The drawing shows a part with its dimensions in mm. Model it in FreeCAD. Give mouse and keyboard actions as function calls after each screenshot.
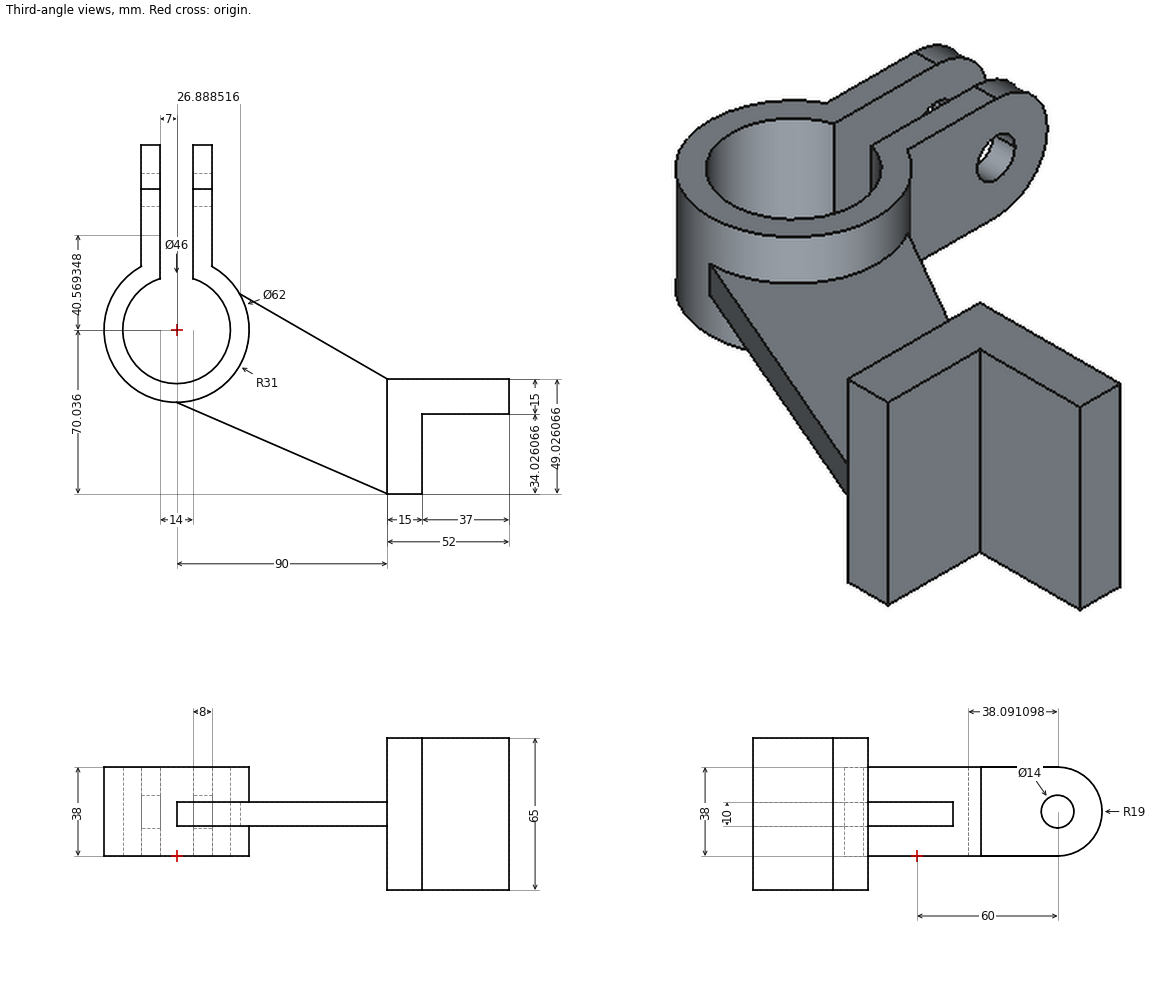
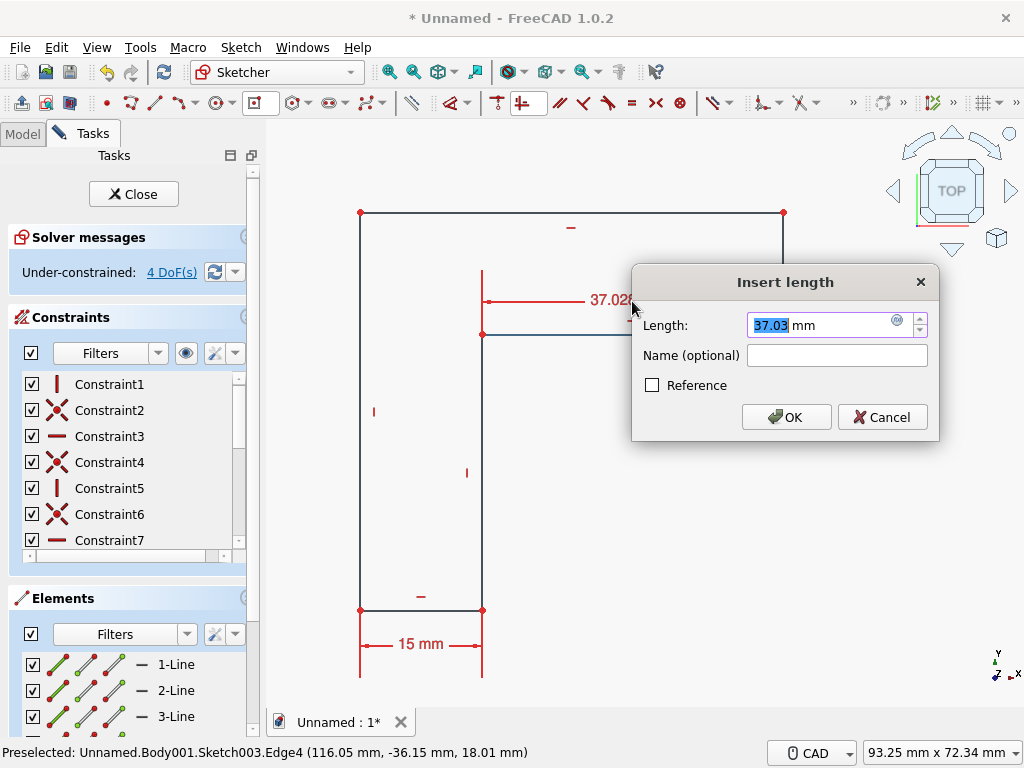
text(37)
key(Return)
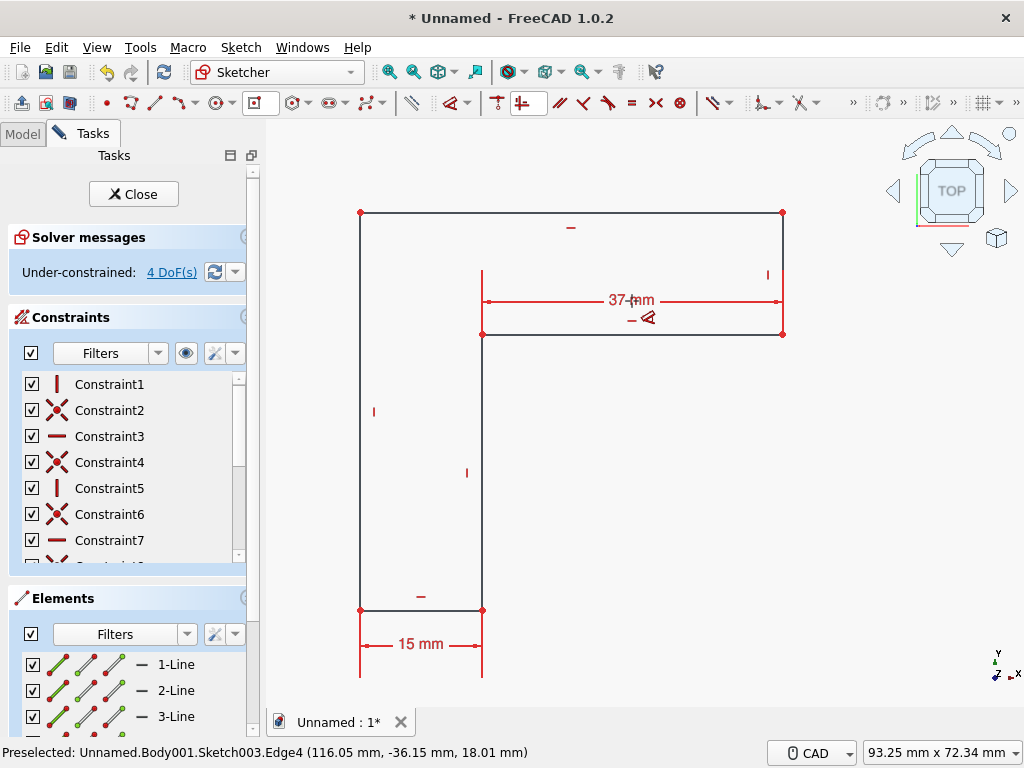
click(783, 298)
click(817, 274)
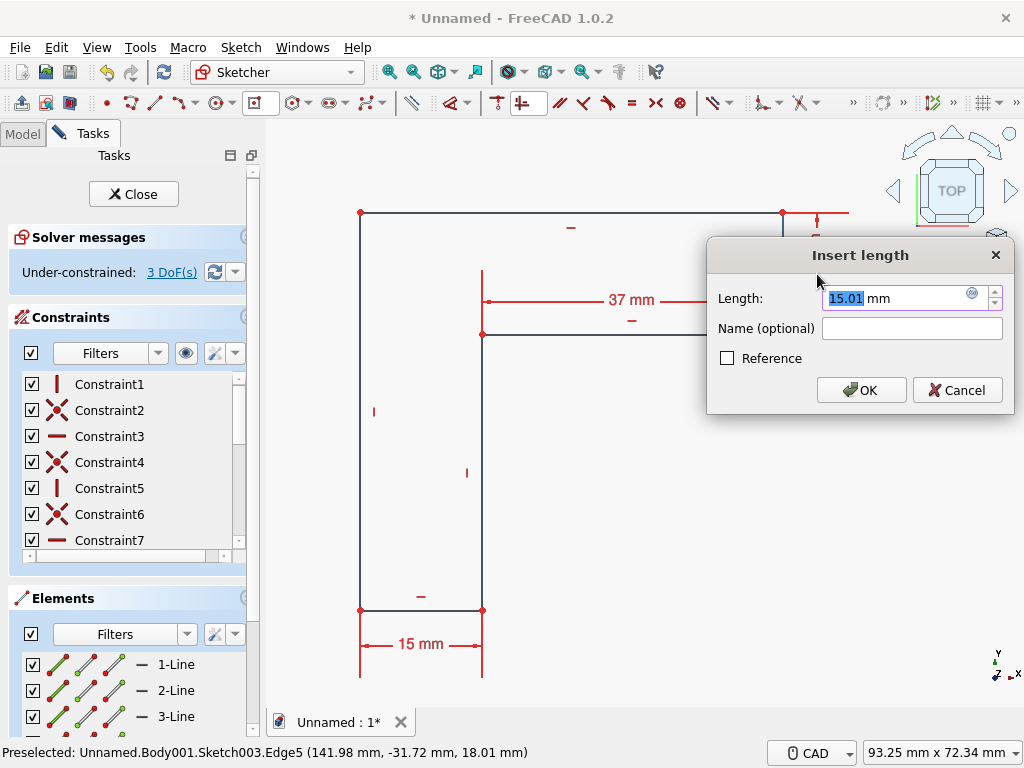
text(15)
key(Return)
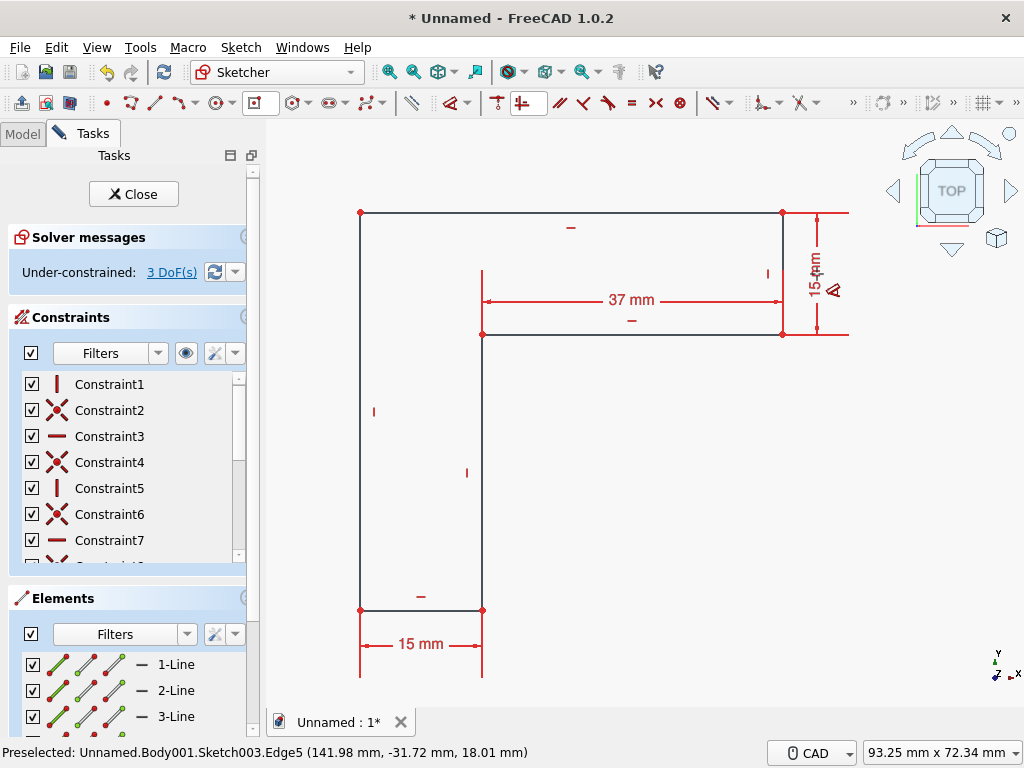
click(360, 213)
click(327, 247)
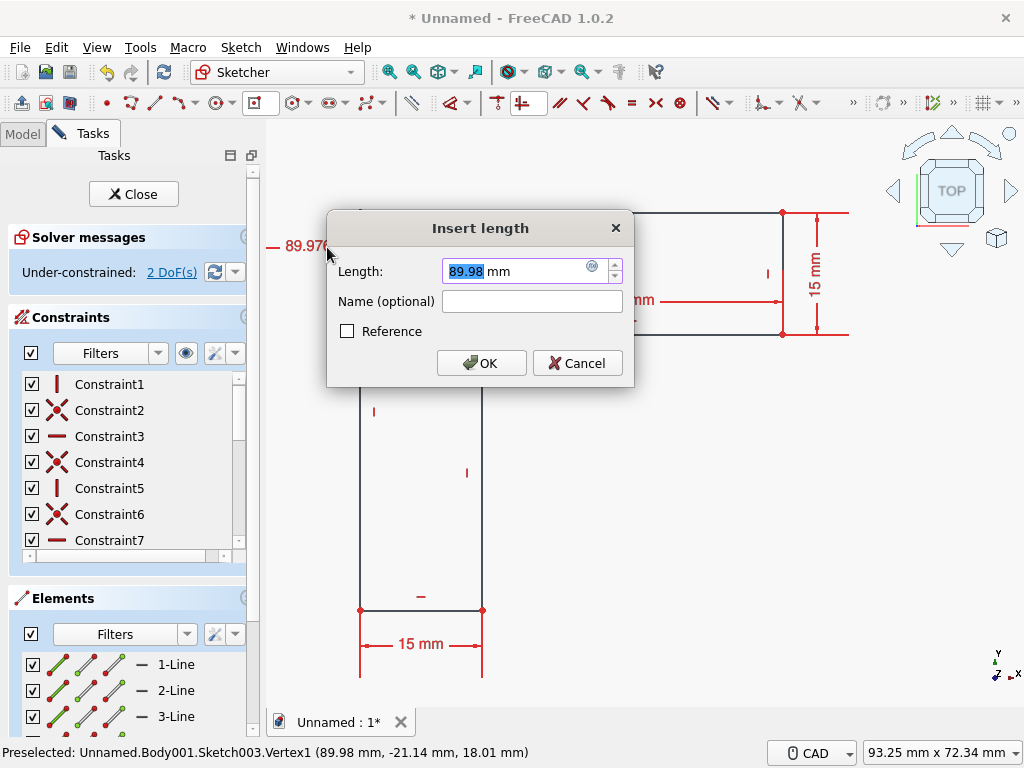
text(90)
key(Return)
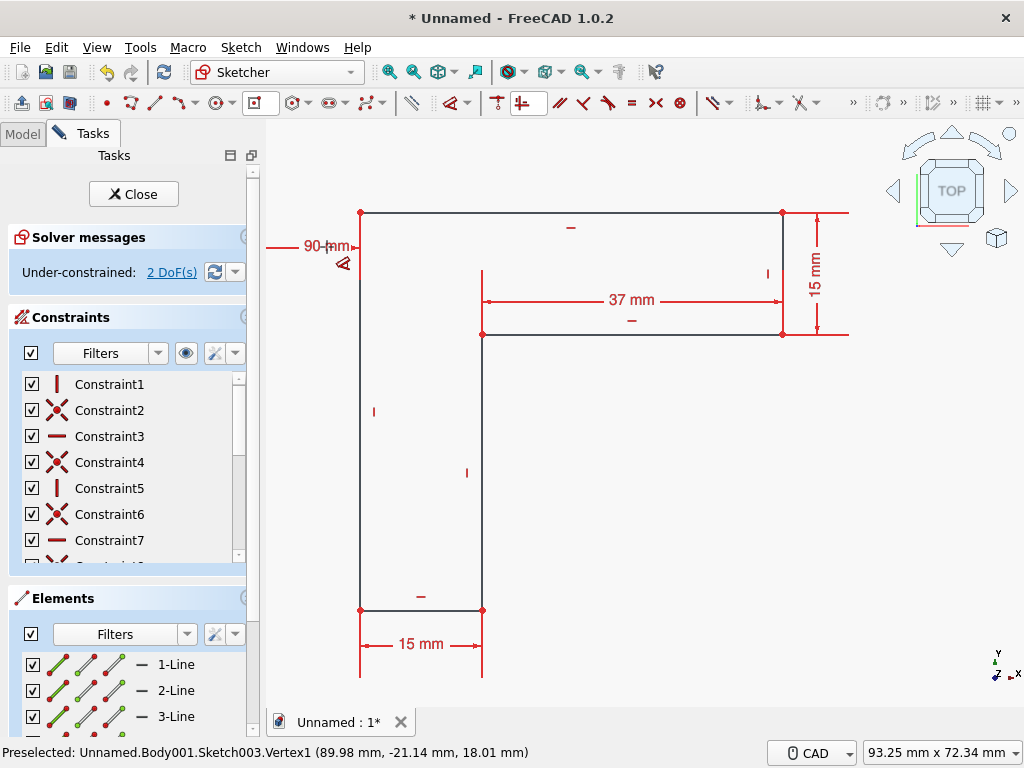
click(360, 611)
click(394, 379)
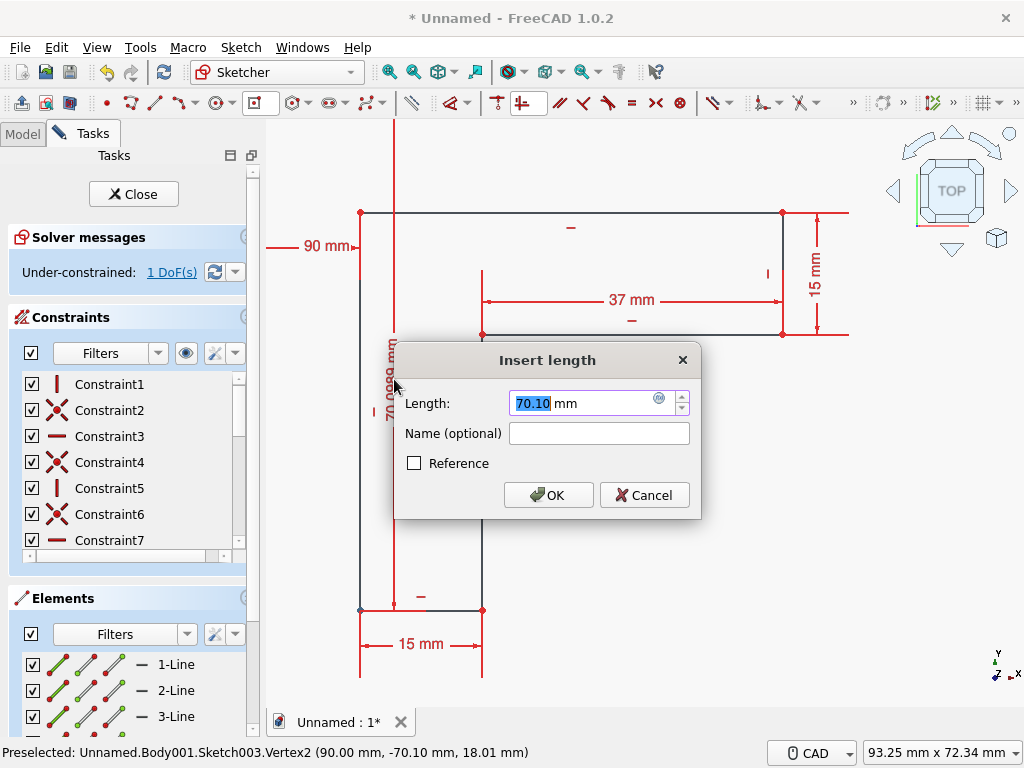
text(70.036)
key(Return)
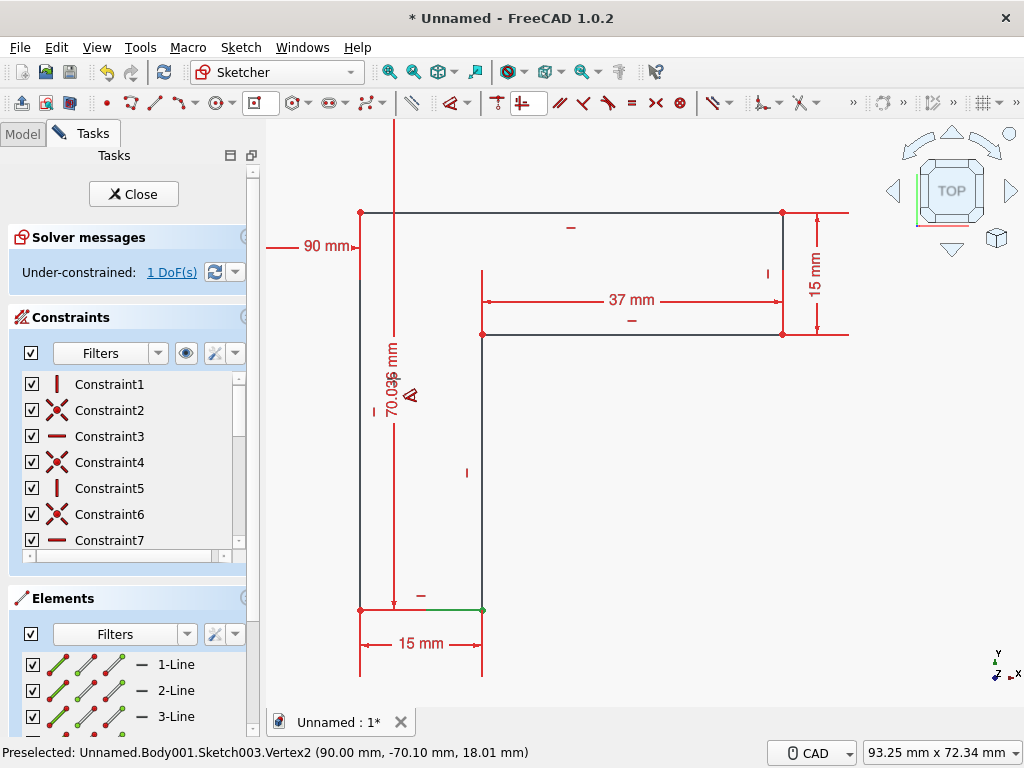
click(360, 332)
click(326, 412)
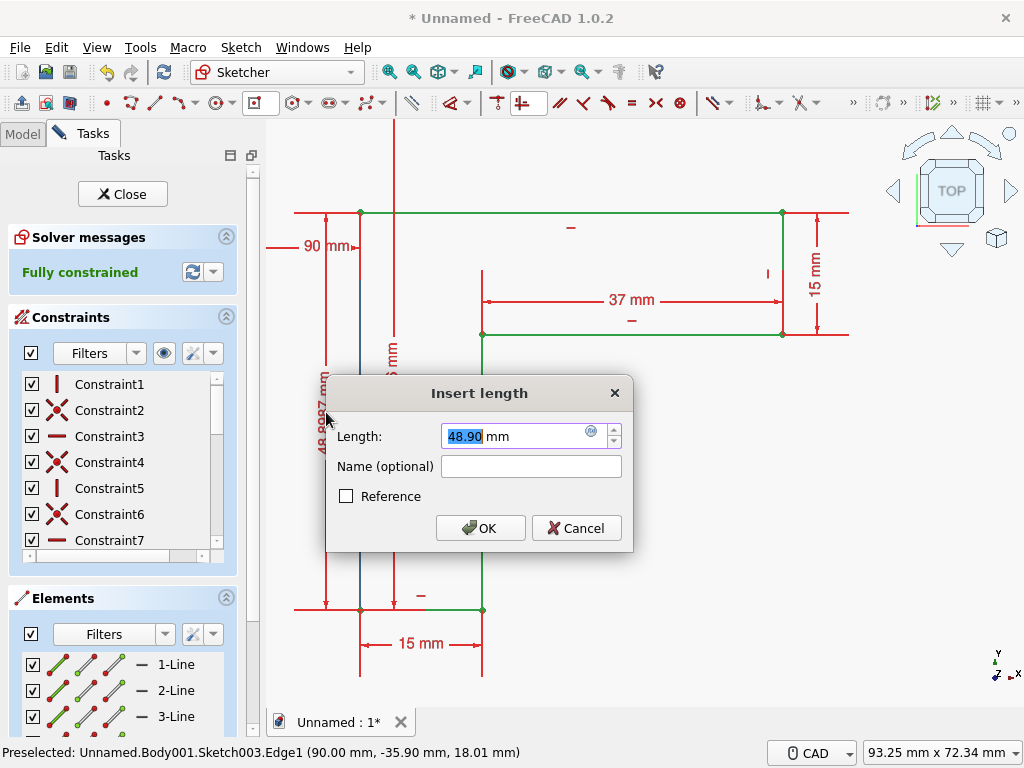
text(49.026066)
key(Return)
key(Escape)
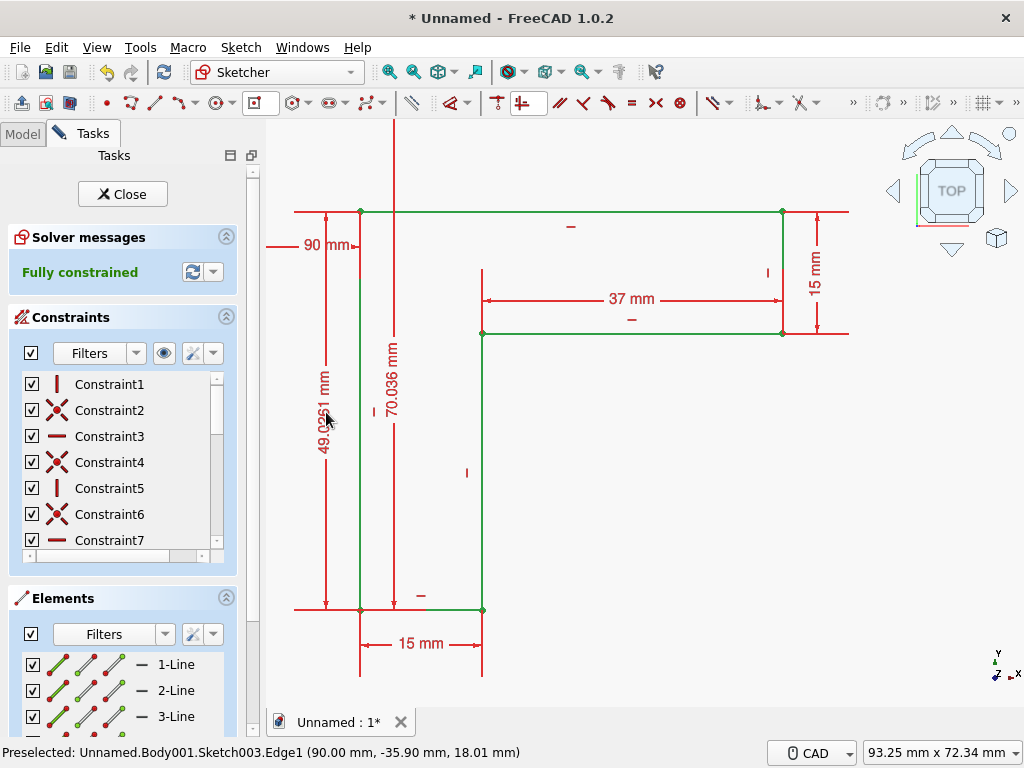
click(123, 194)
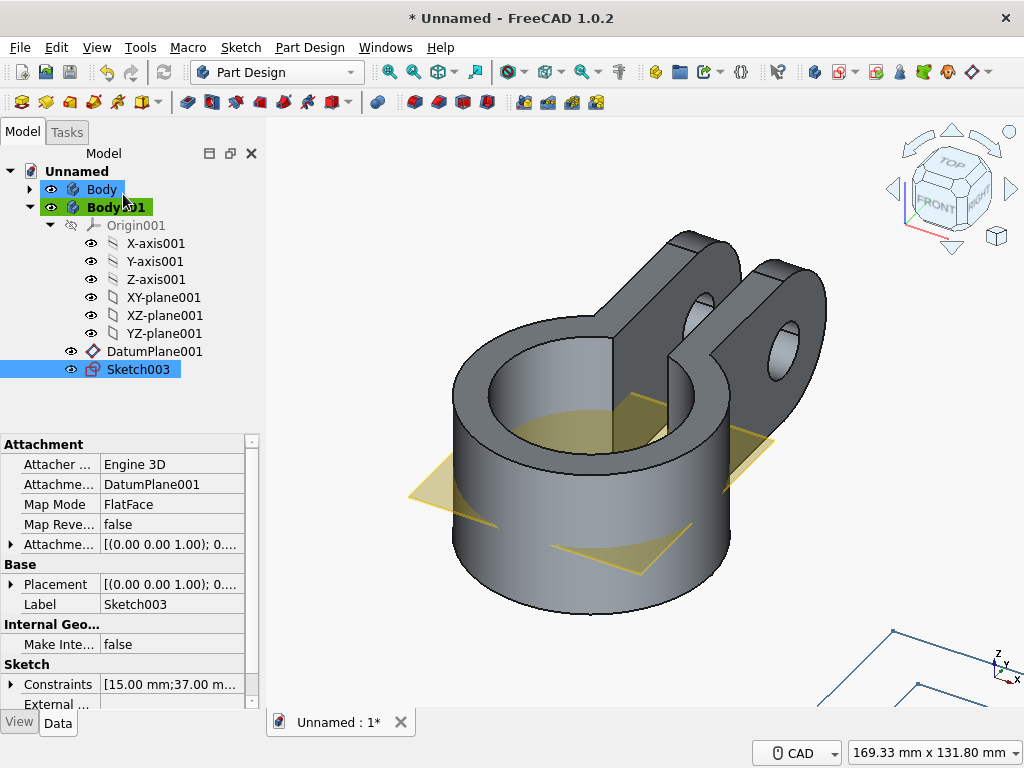
click(22, 102)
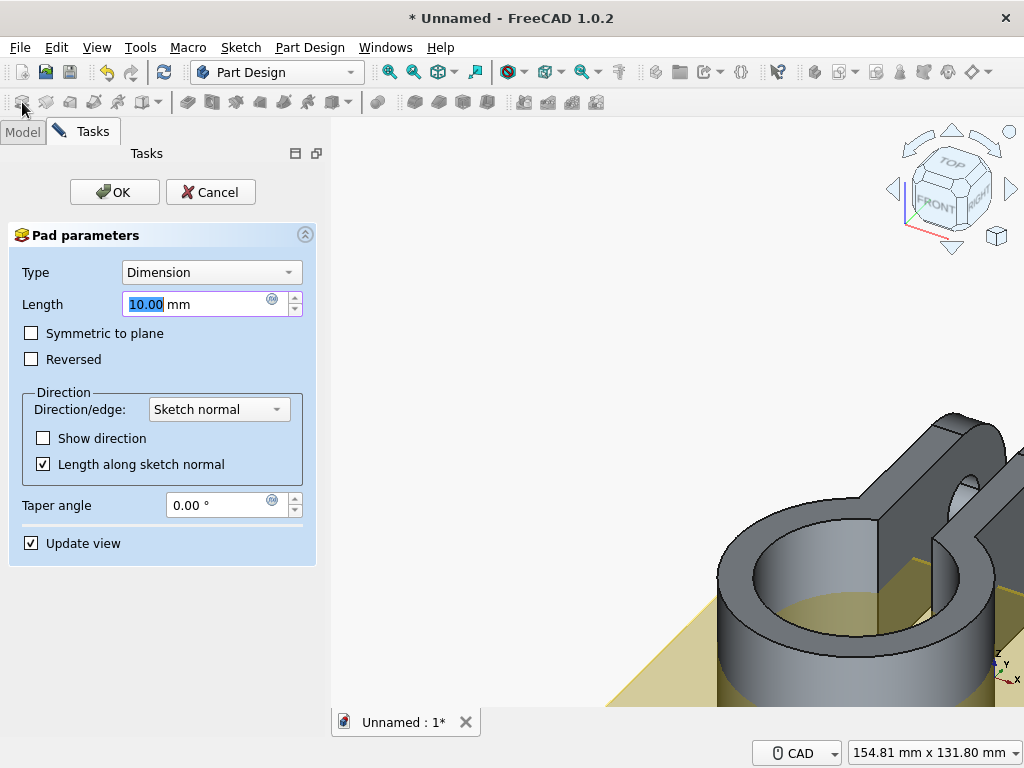
text(65)
key(Tab)